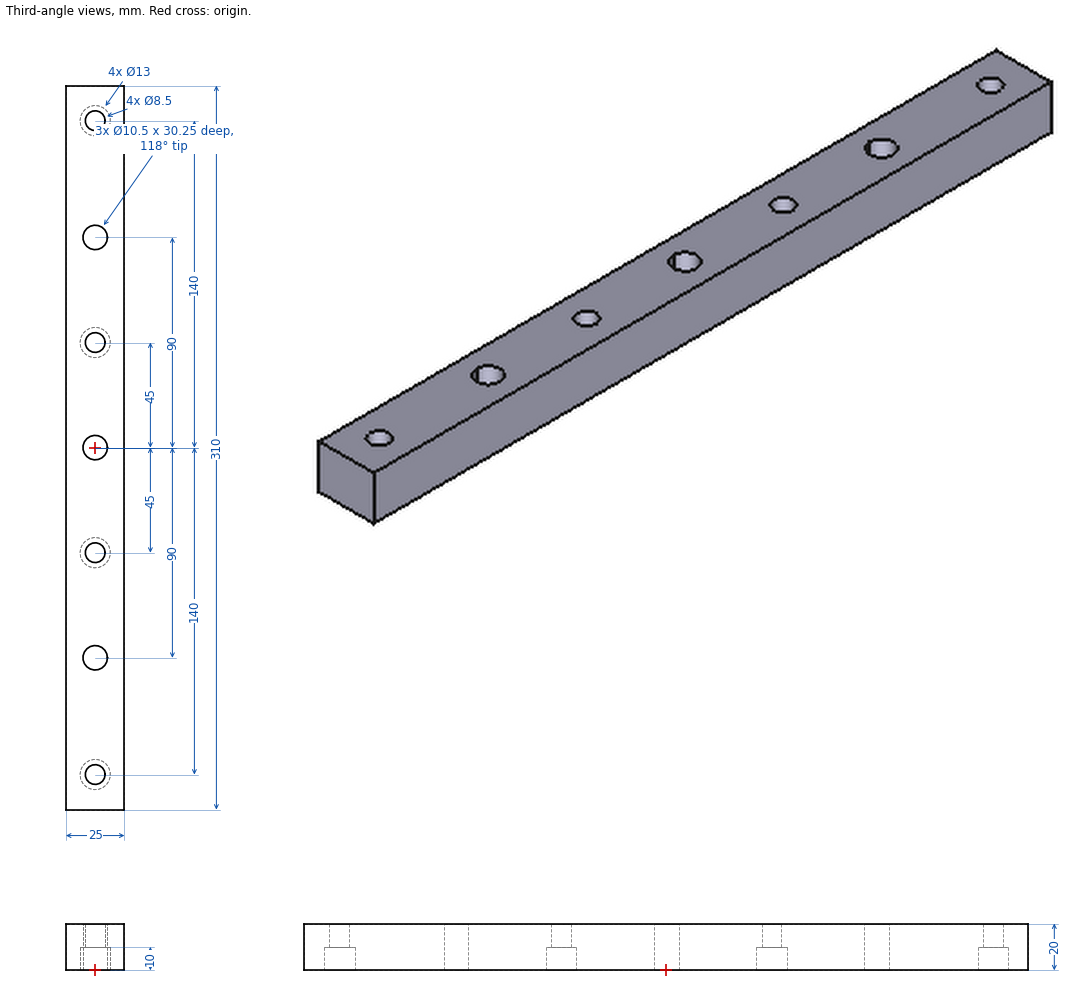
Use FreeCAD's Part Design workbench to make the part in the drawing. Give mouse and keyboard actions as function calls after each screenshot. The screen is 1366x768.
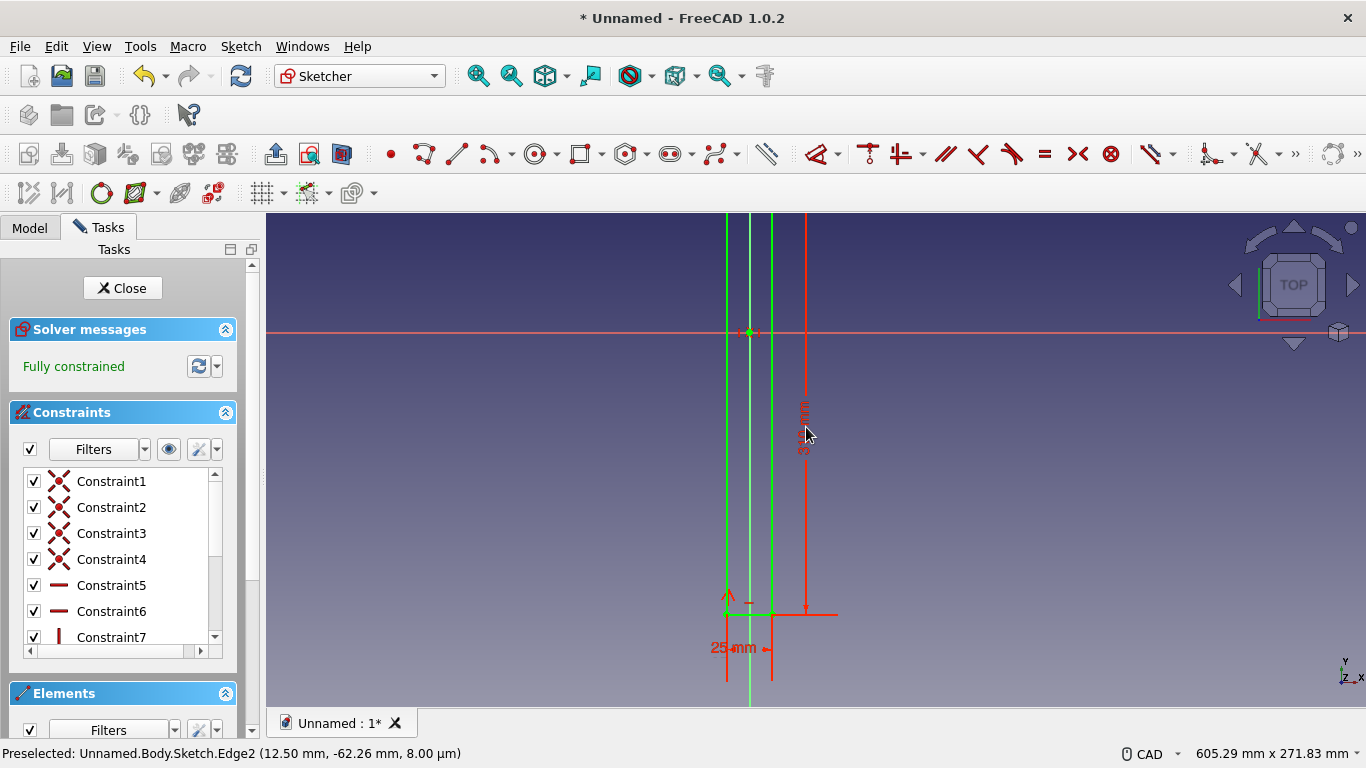
click(123, 288)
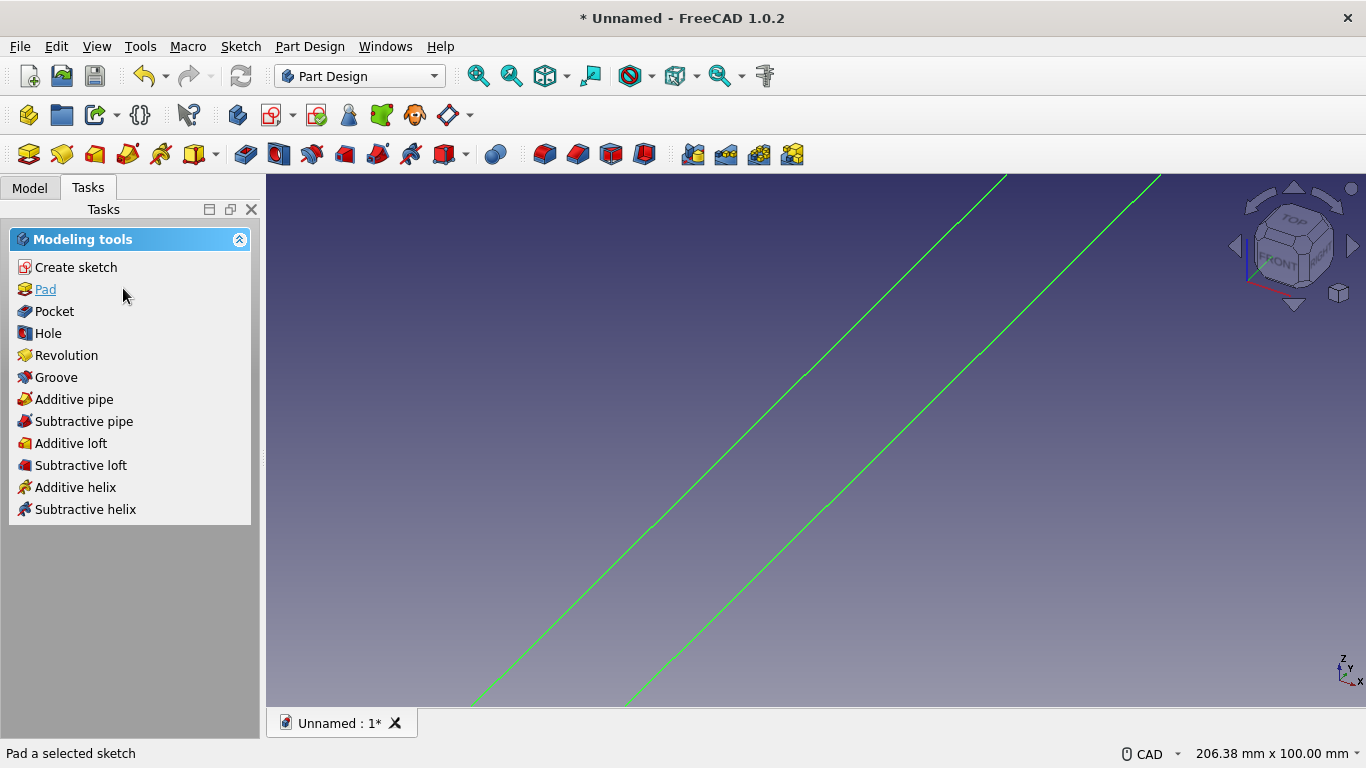
click(29, 154)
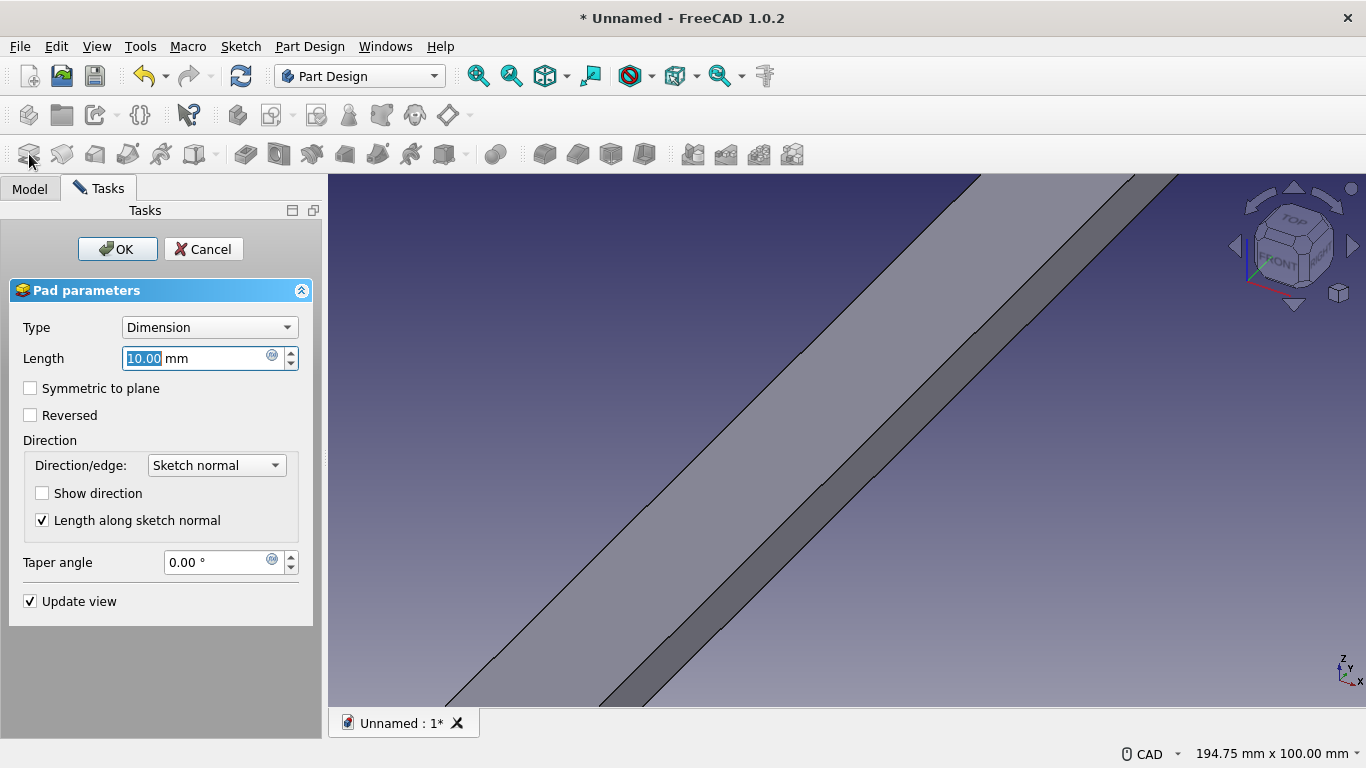
text(20)
key(Tab)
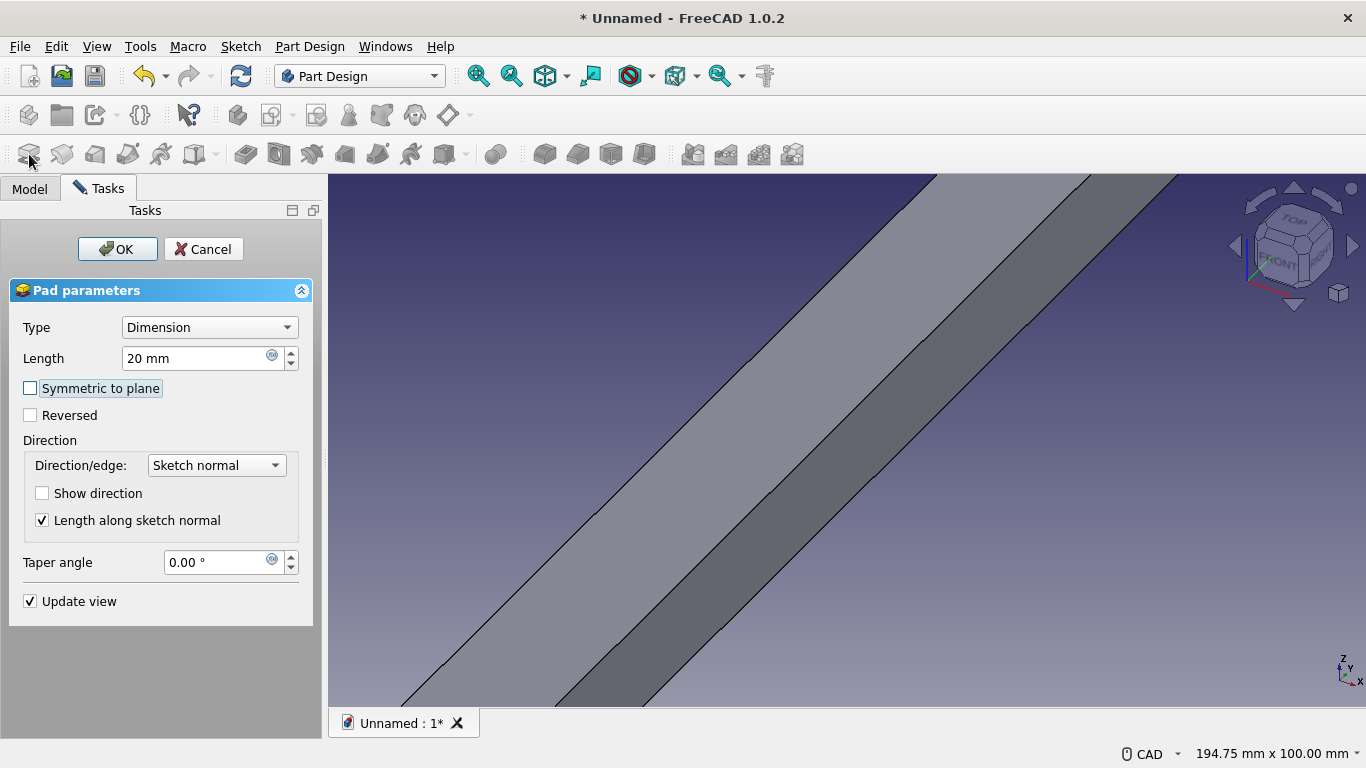
click(118, 249)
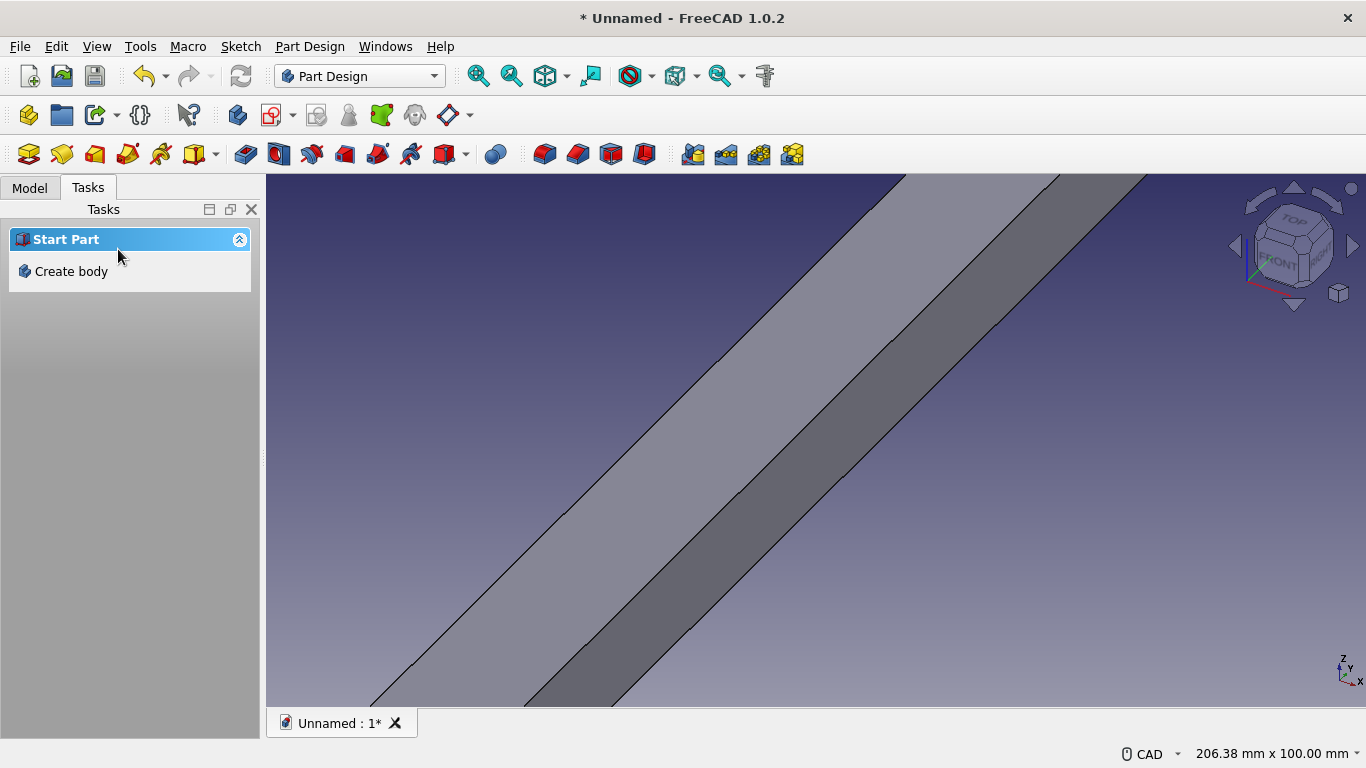
click(479, 76)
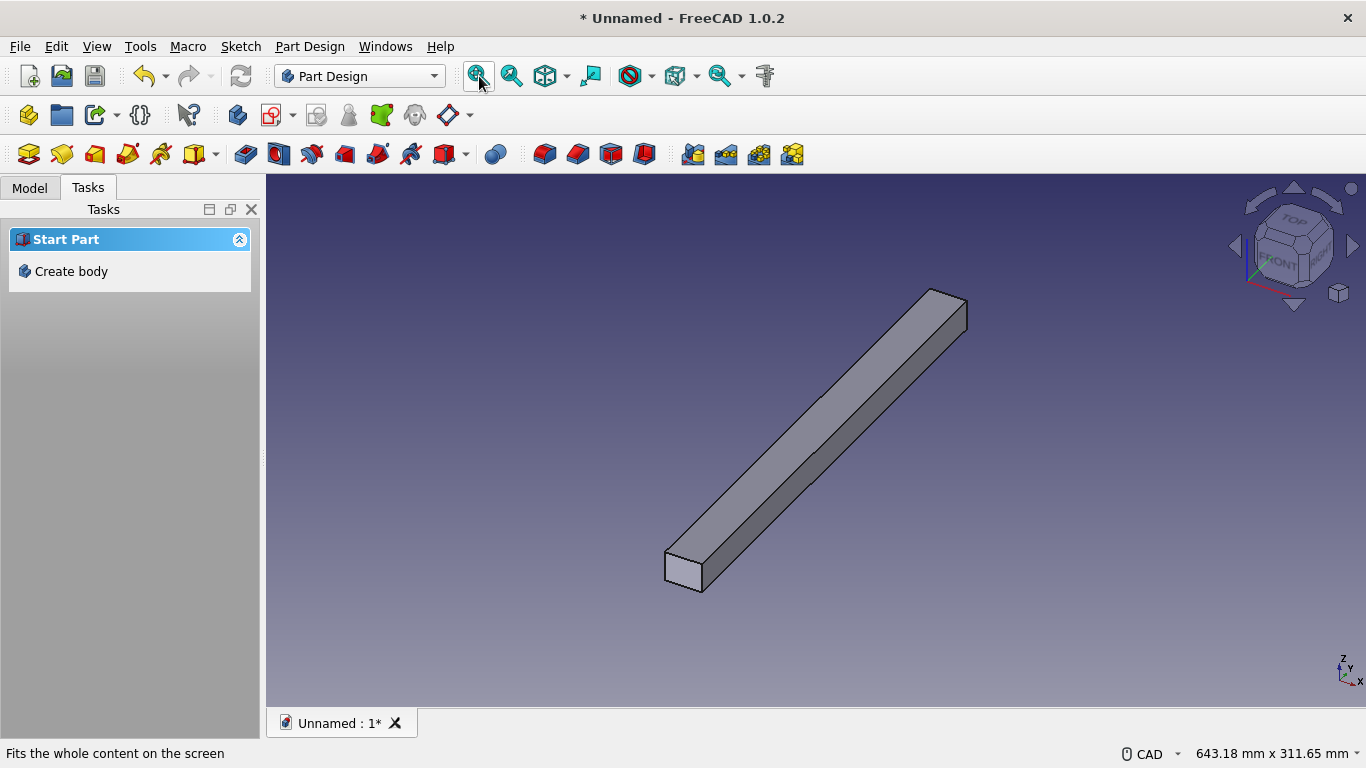
click(930, 313)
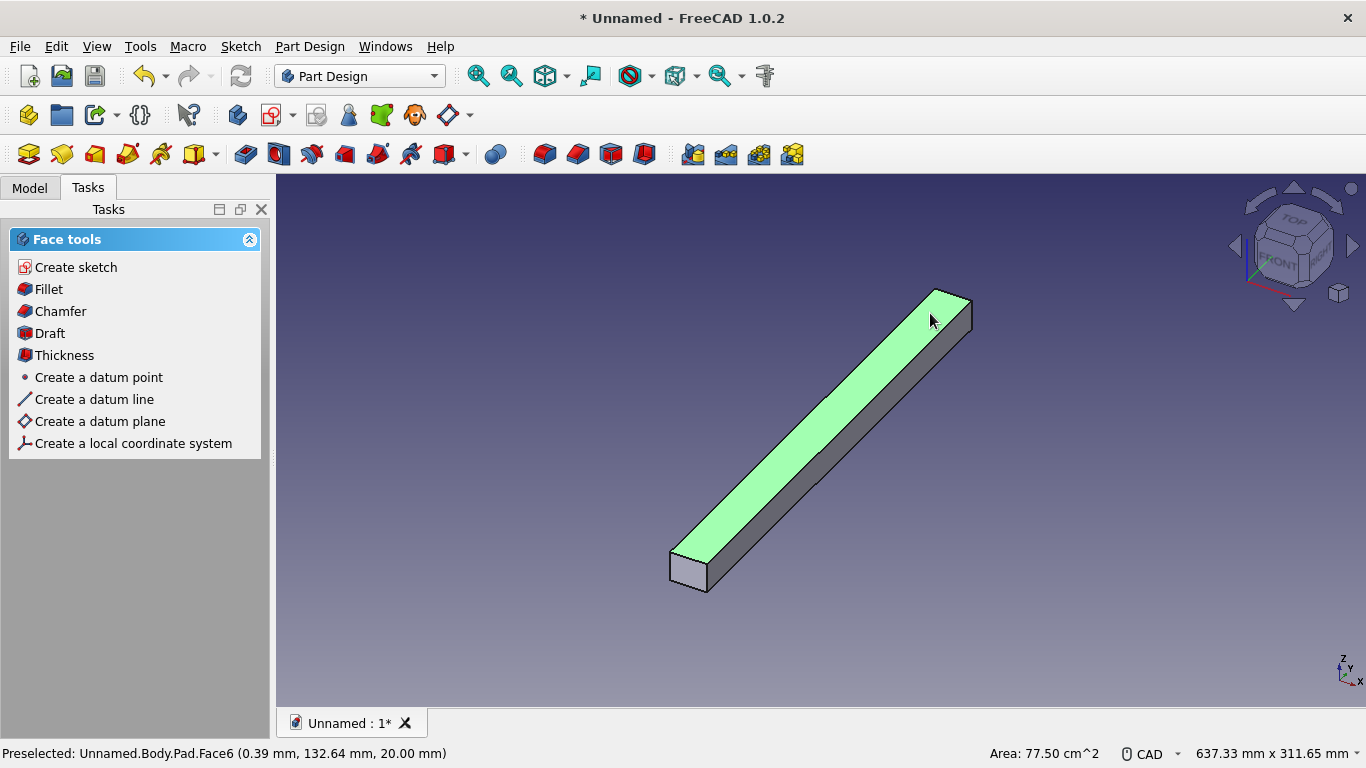
click(270, 116)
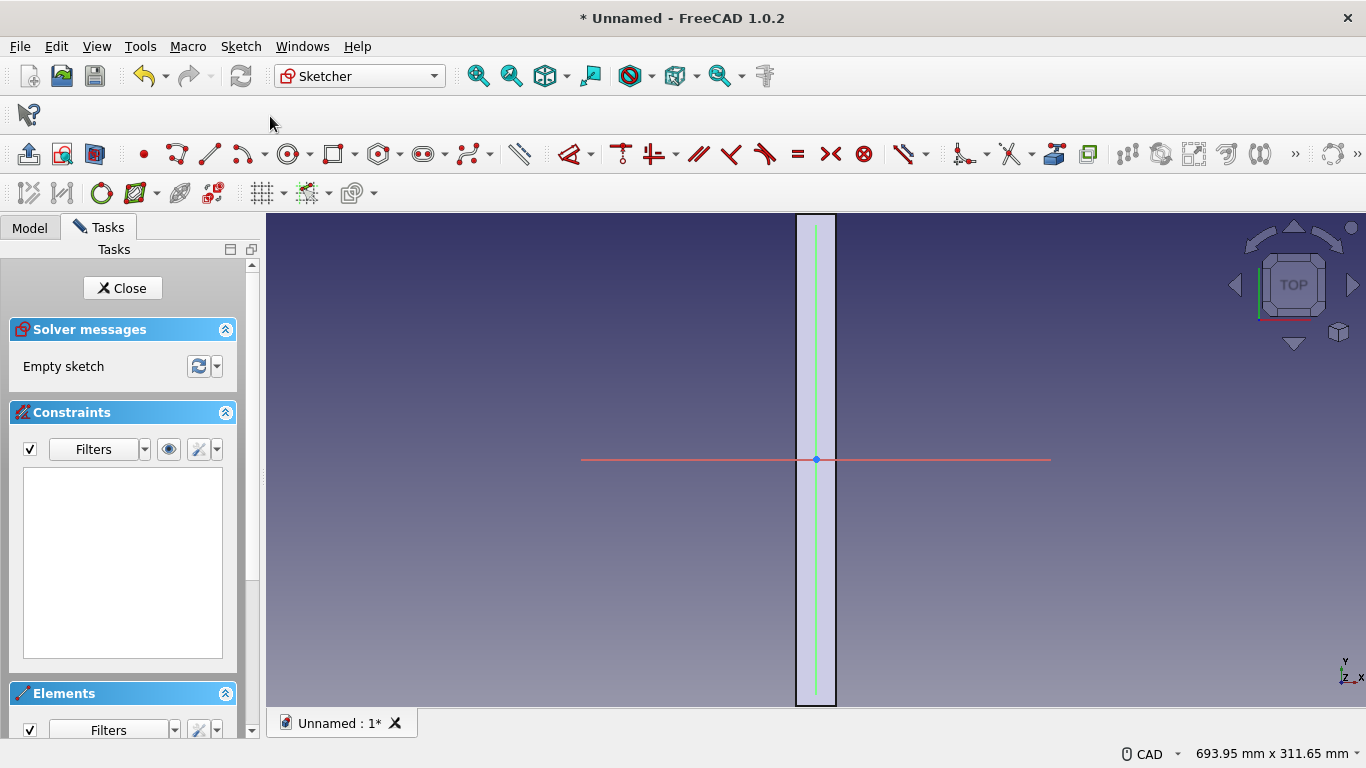
scroll(608, 460, down, 2)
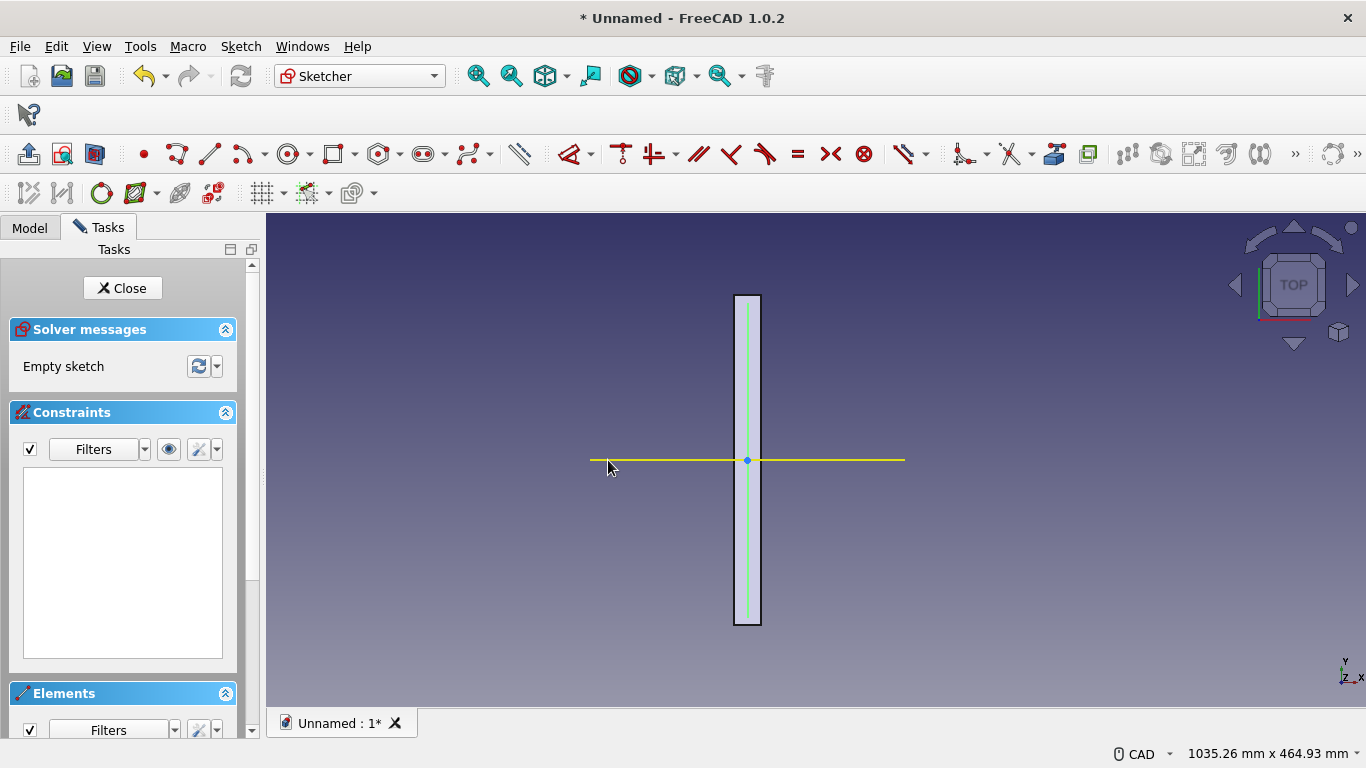
key(g)
key(c)